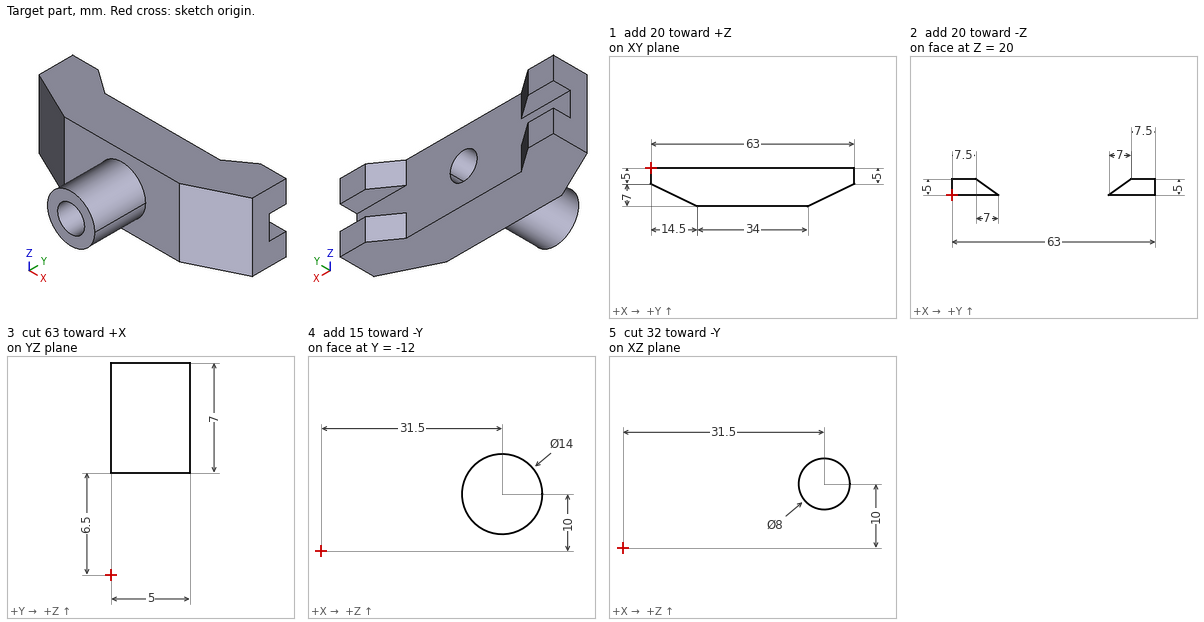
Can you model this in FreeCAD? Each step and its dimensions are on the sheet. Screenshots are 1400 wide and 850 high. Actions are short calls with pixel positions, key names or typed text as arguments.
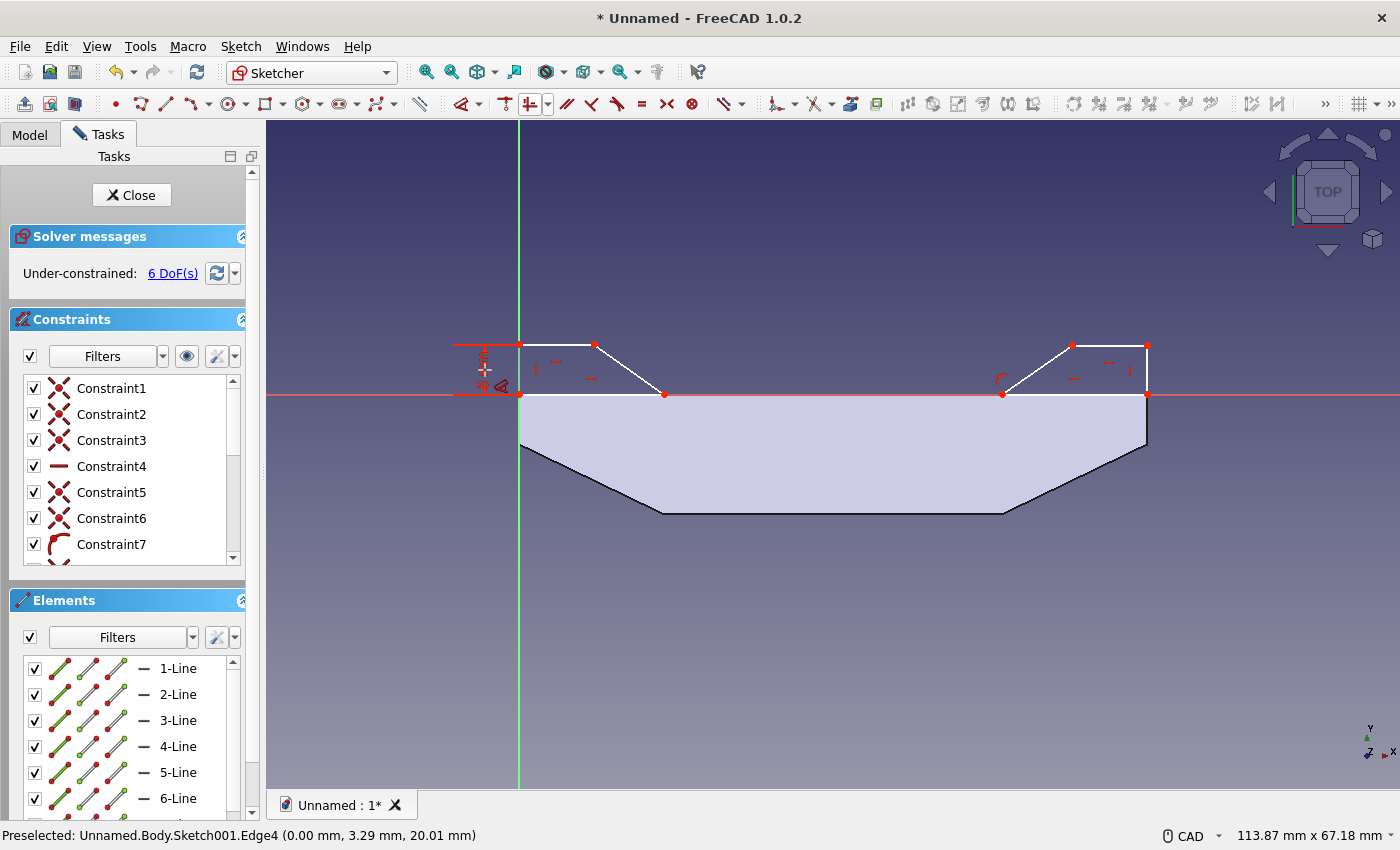
click(1147, 380)
click(1181, 370)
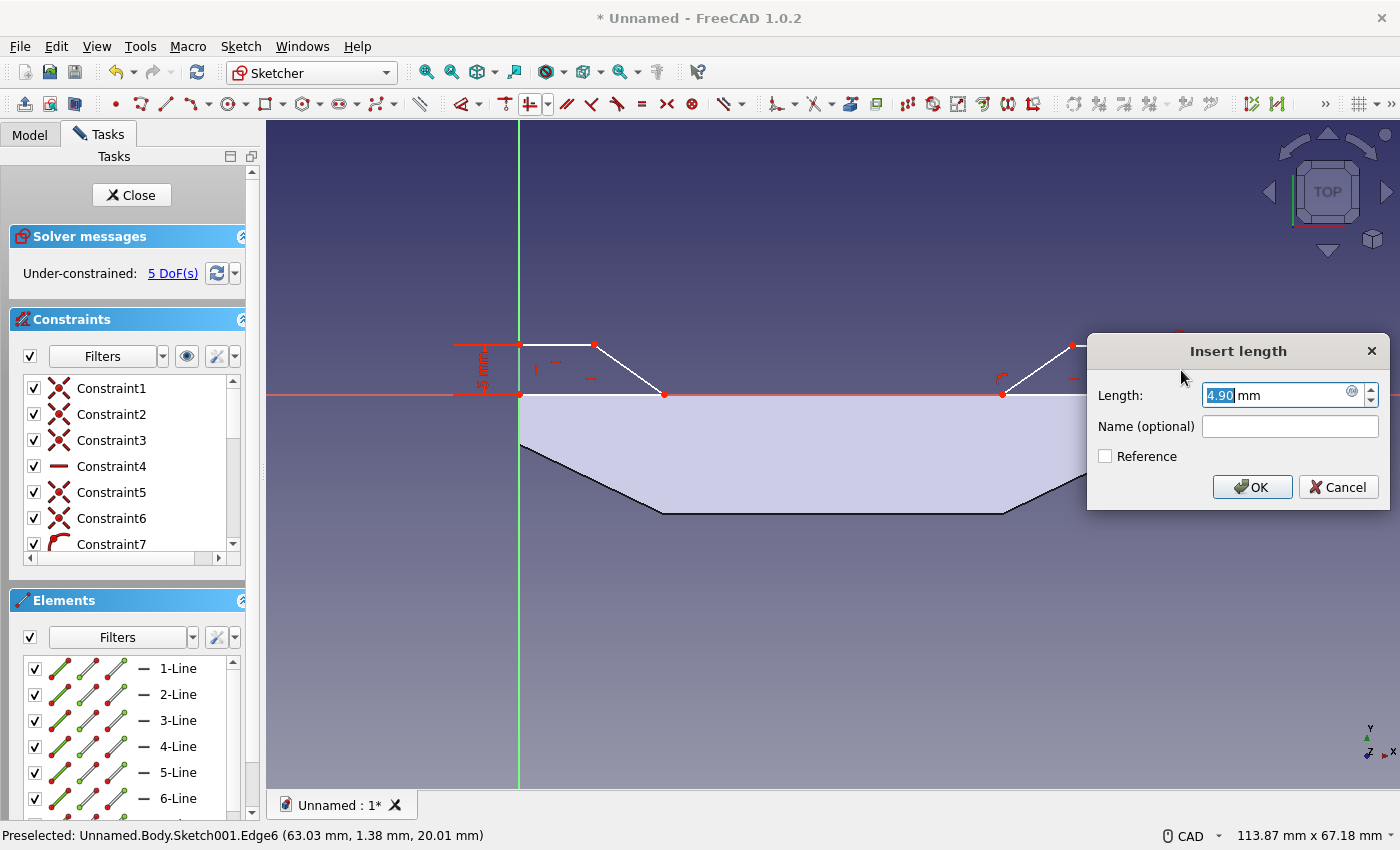
text(5)
key(Return)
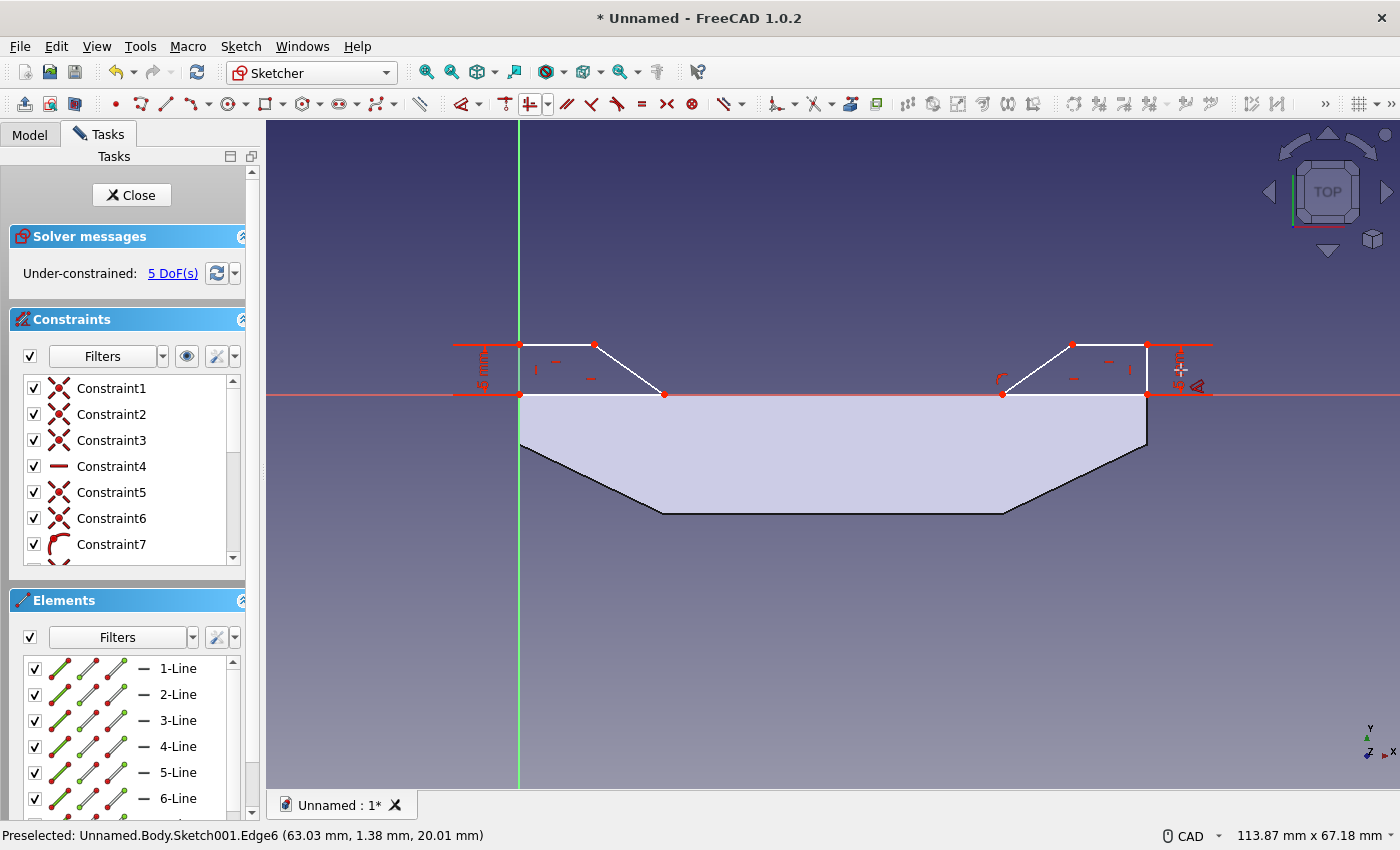
click(643, 380)
click(629, 429)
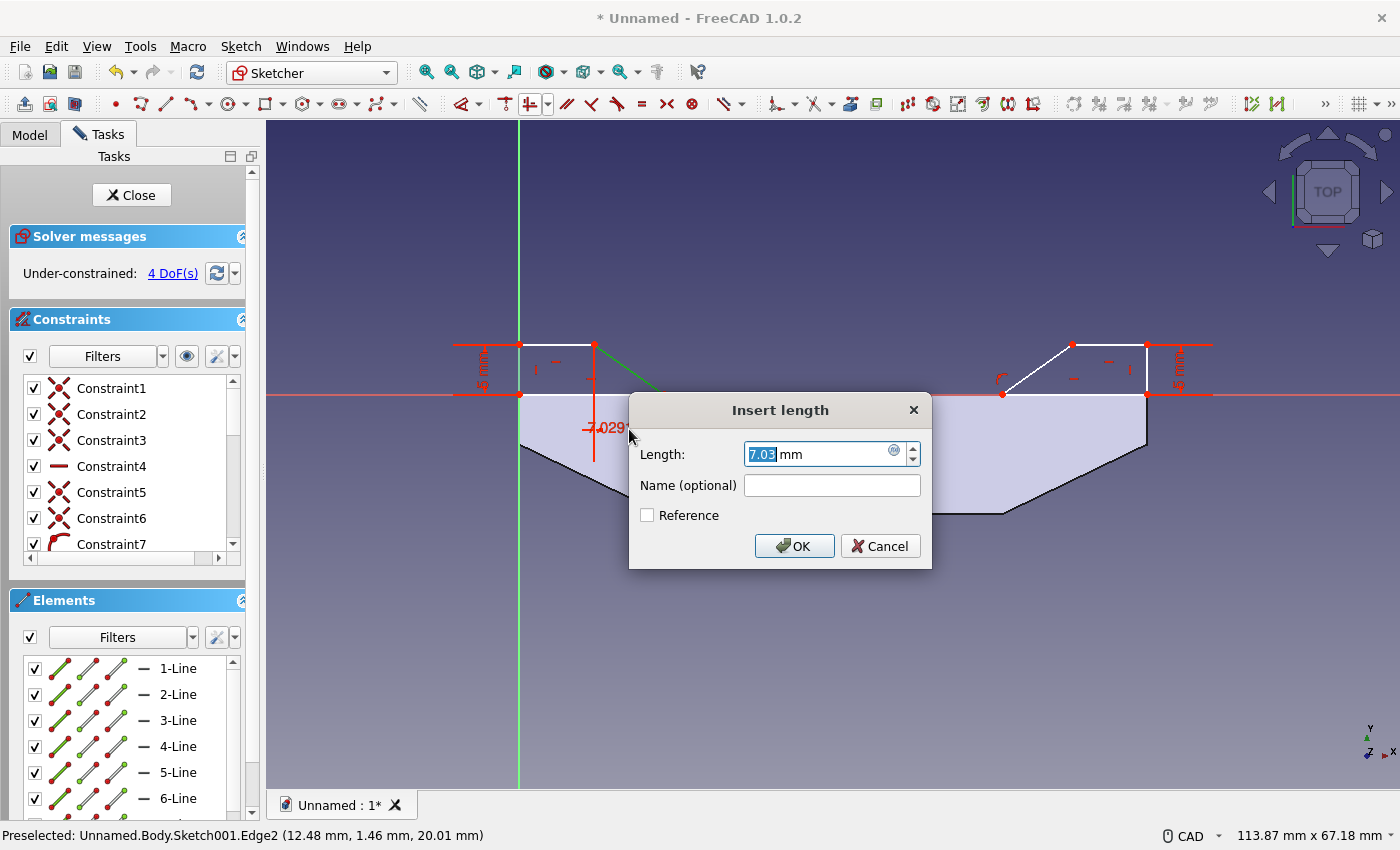
text(7)
key(Return)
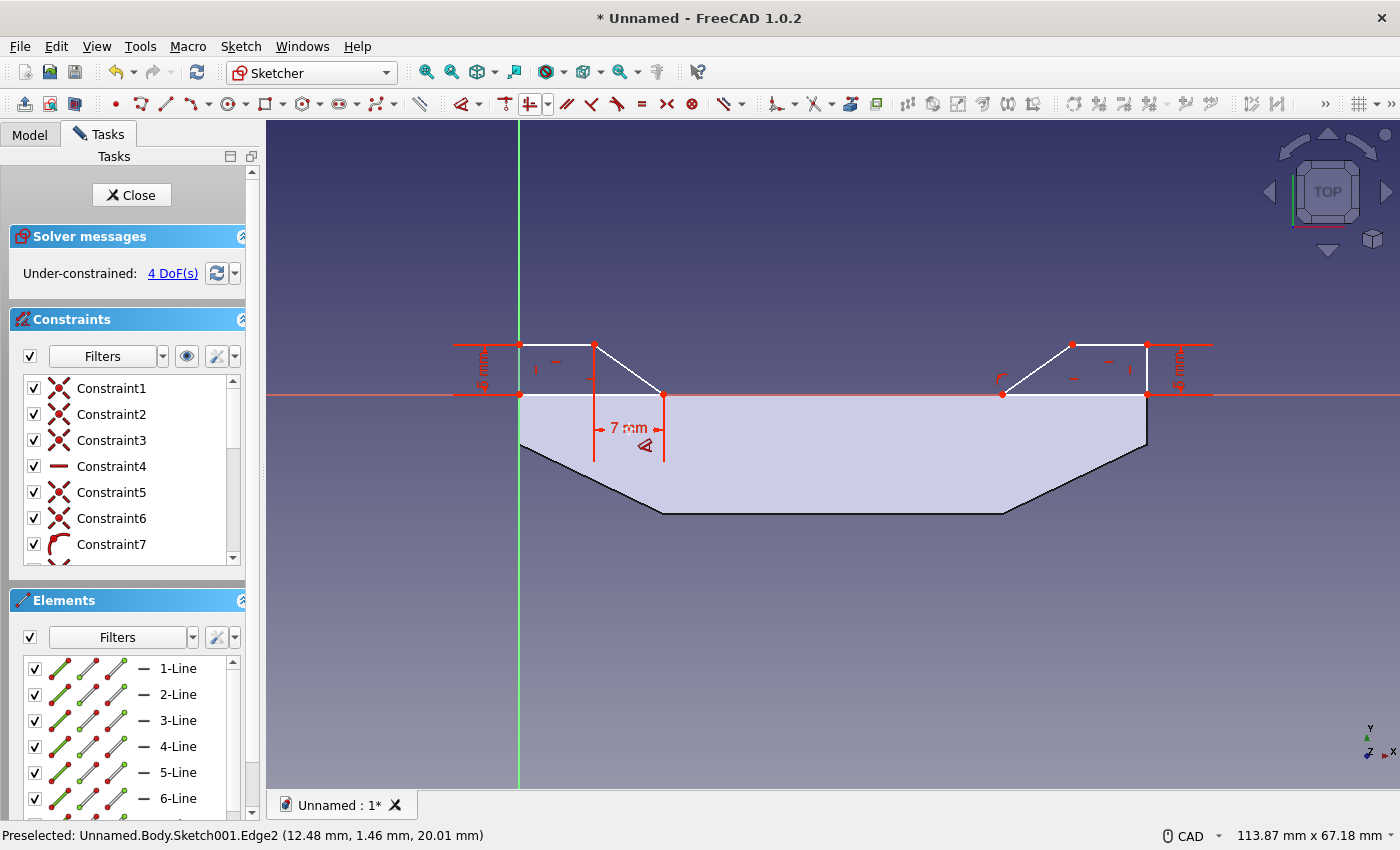
click(1051, 360)
click(1037, 429)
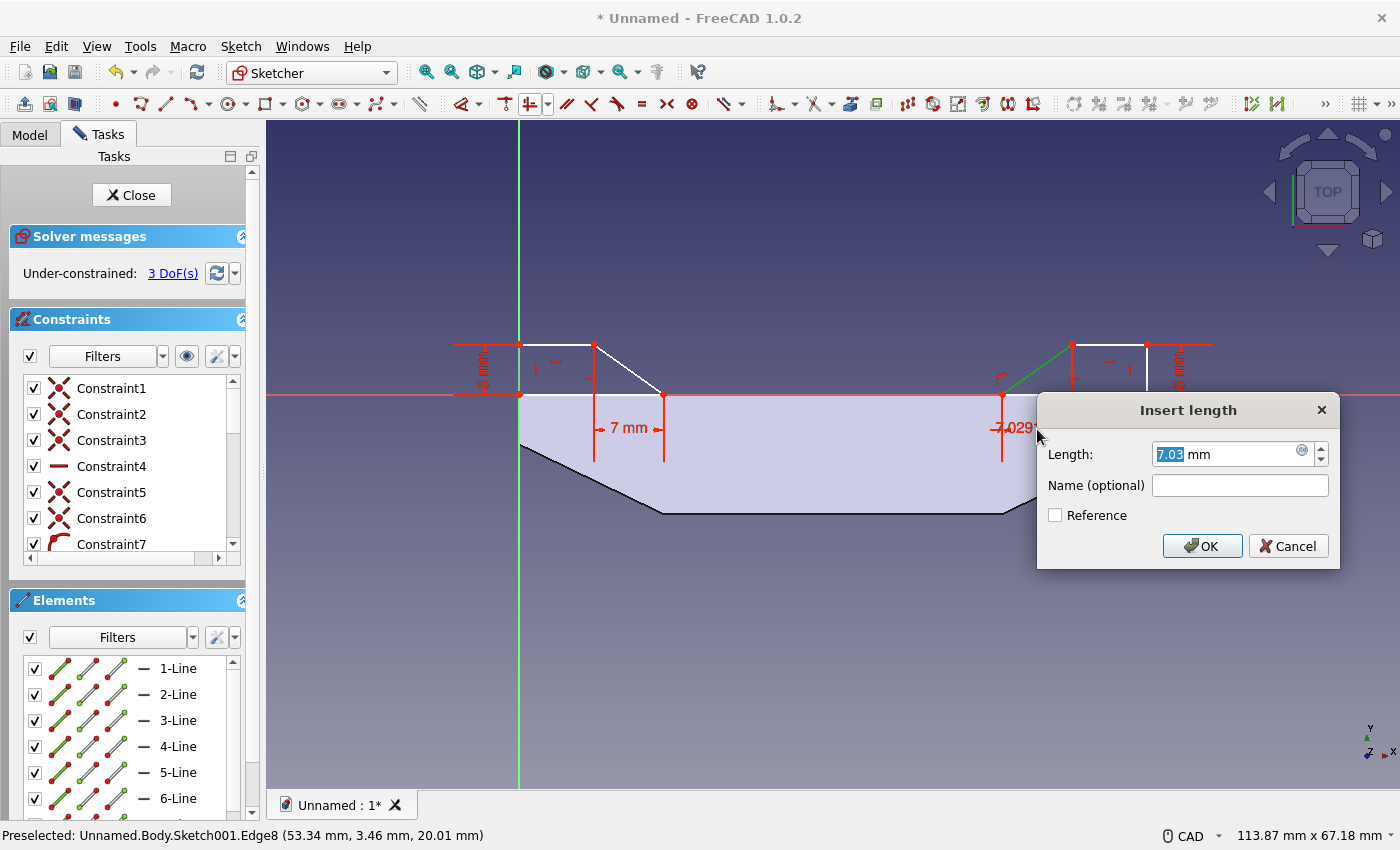
text(7)
key(Return)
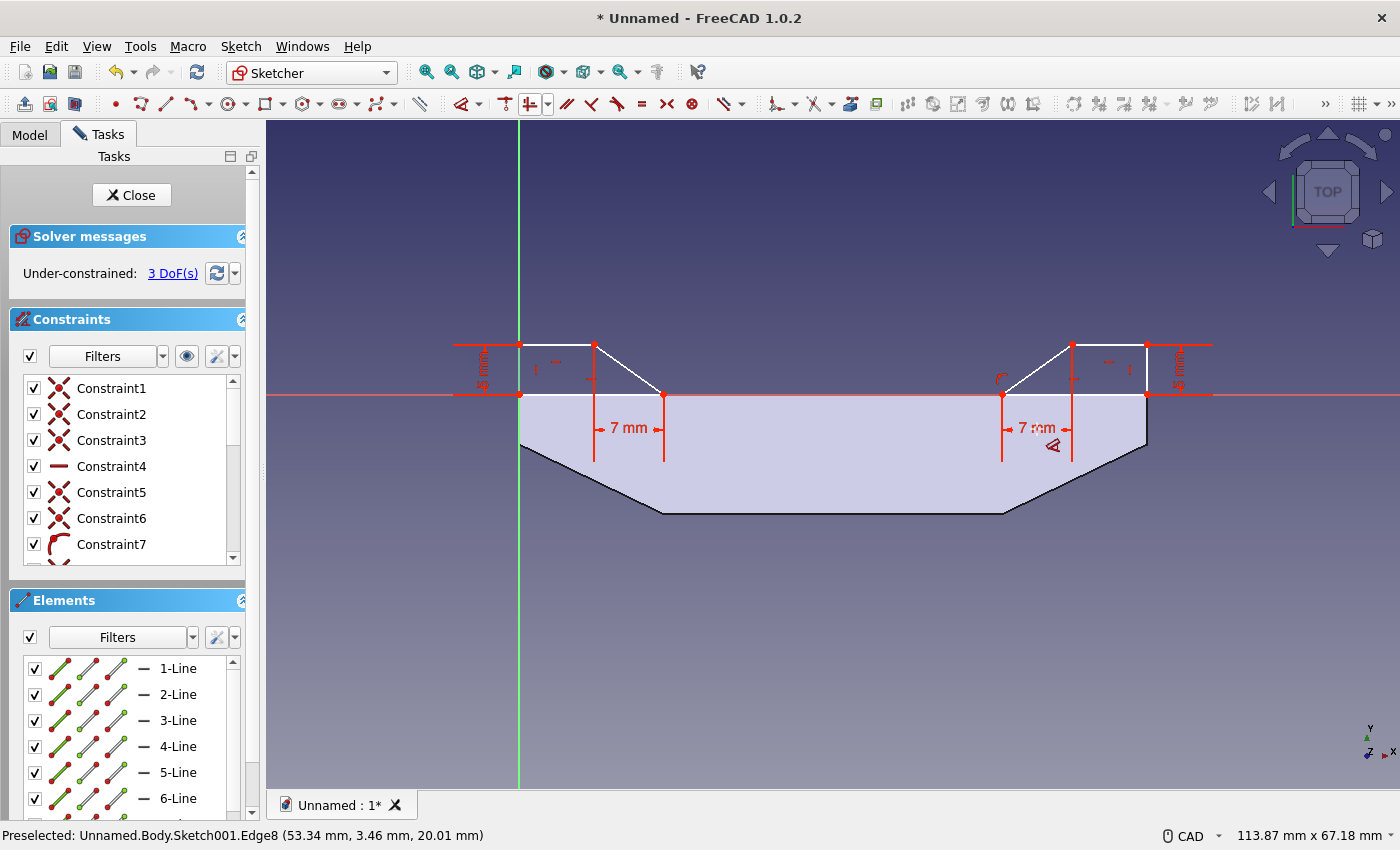
click(572, 345)
click(557, 311)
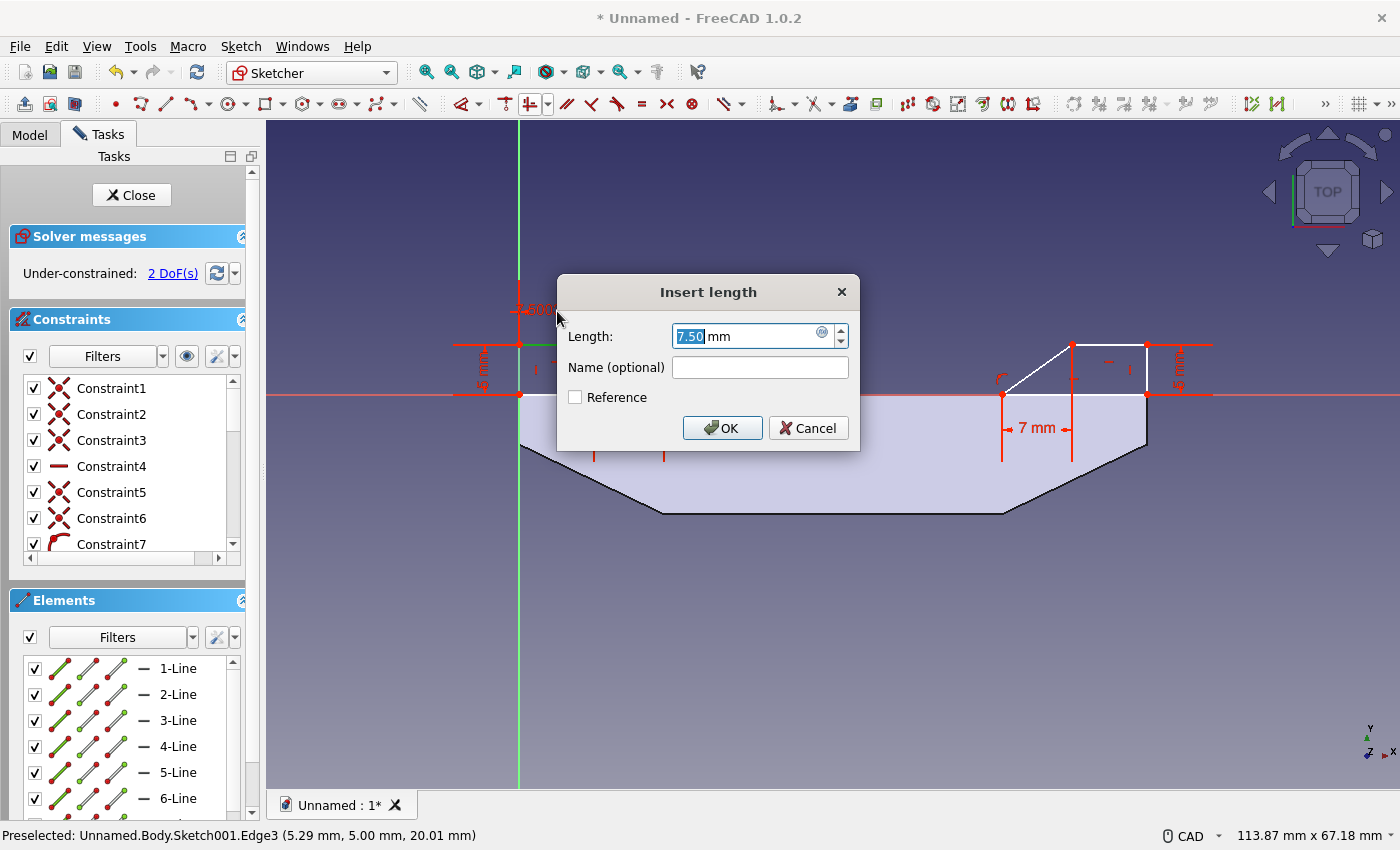
text(7.5)
key(Return)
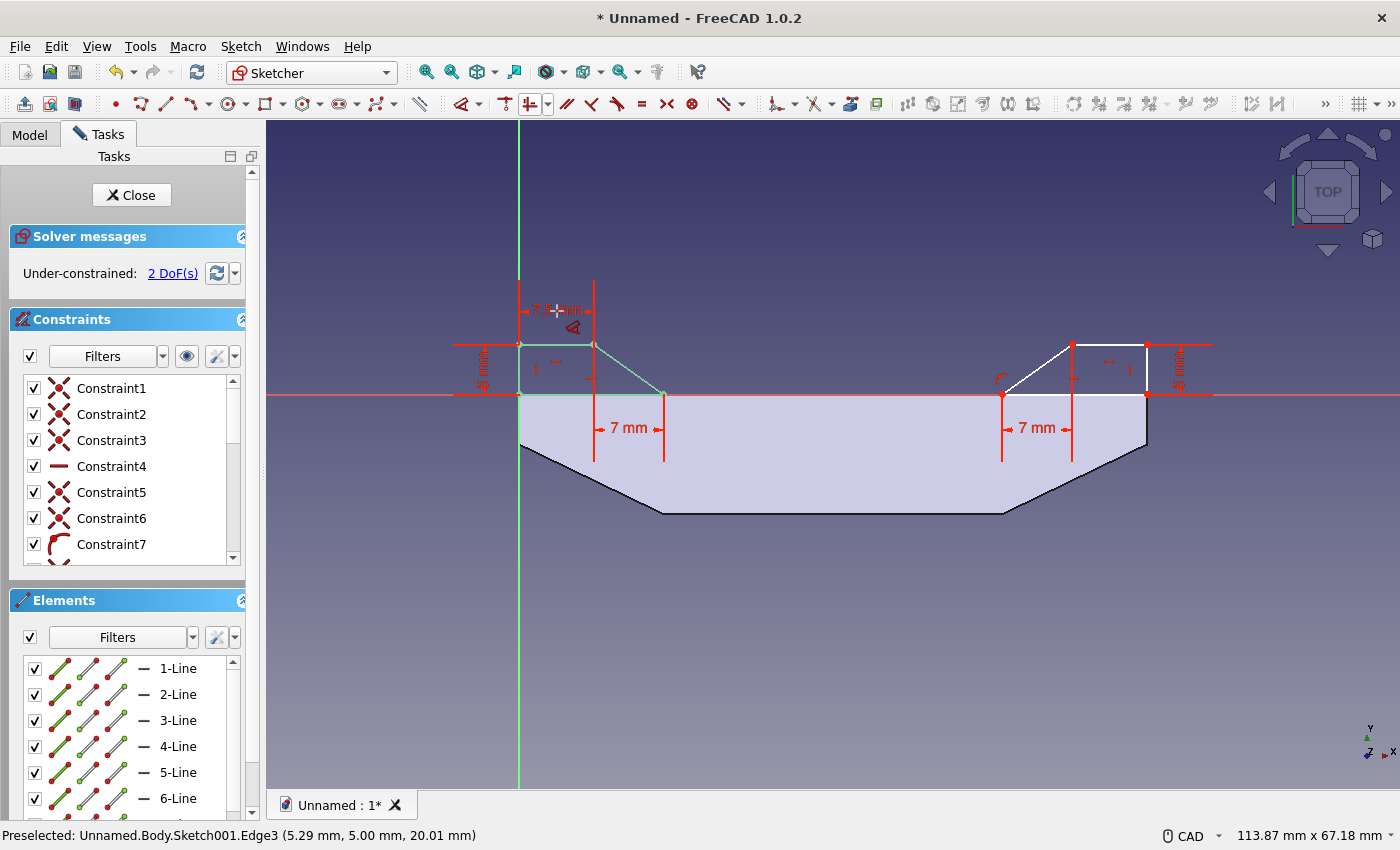
click(1125, 345)
click(1109, 311)